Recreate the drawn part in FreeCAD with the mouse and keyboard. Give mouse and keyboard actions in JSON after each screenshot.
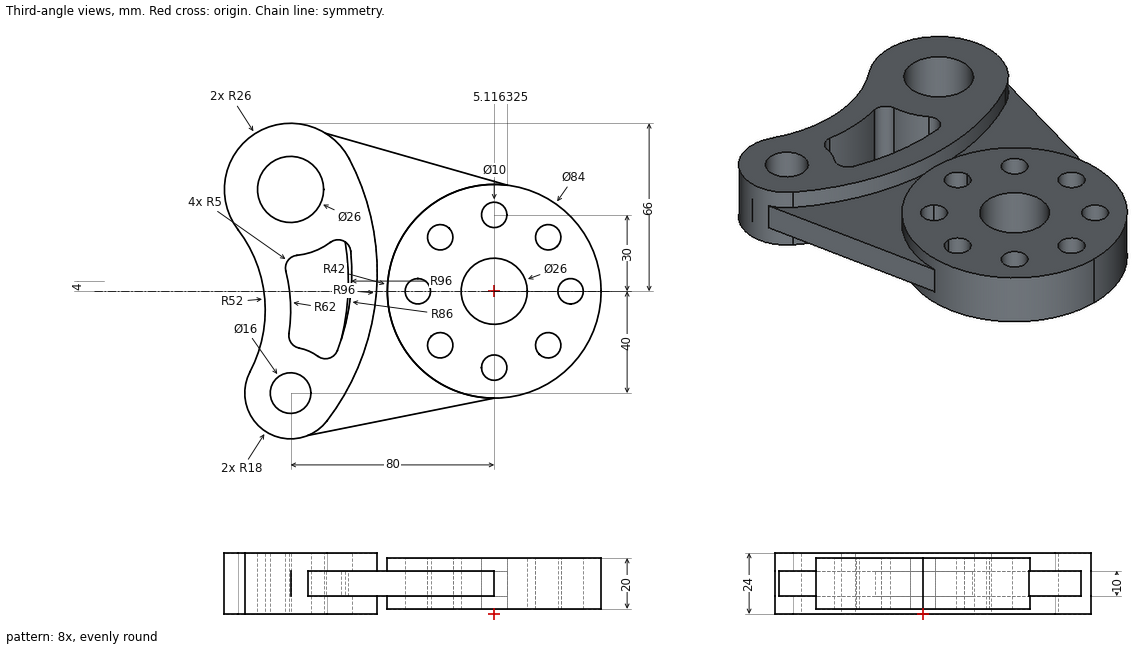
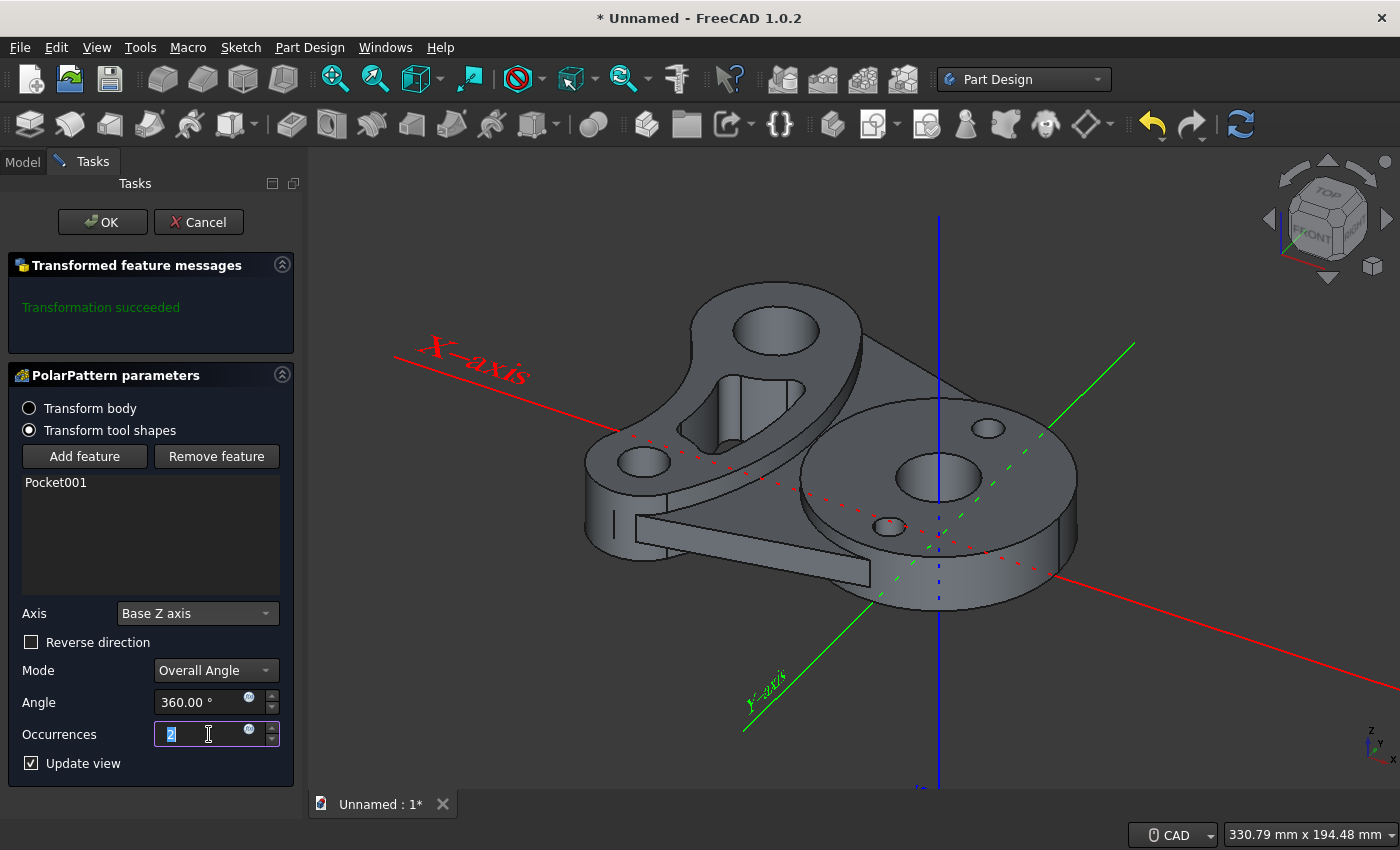
{"action": "type", "text": "8"}
{"action": "key", "text": "Tab"}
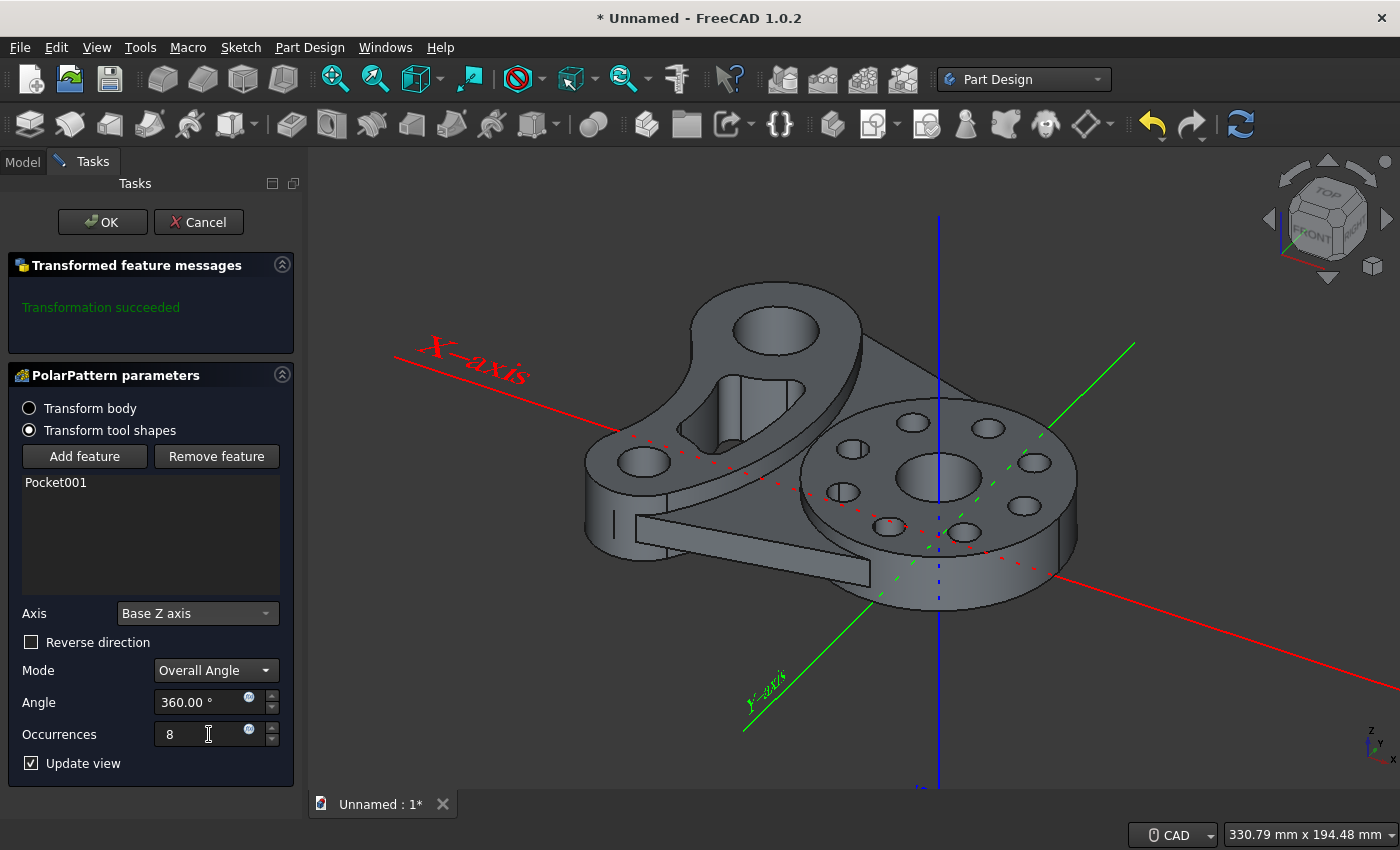
{"action": "left_click", "coordinate": [103, 222]}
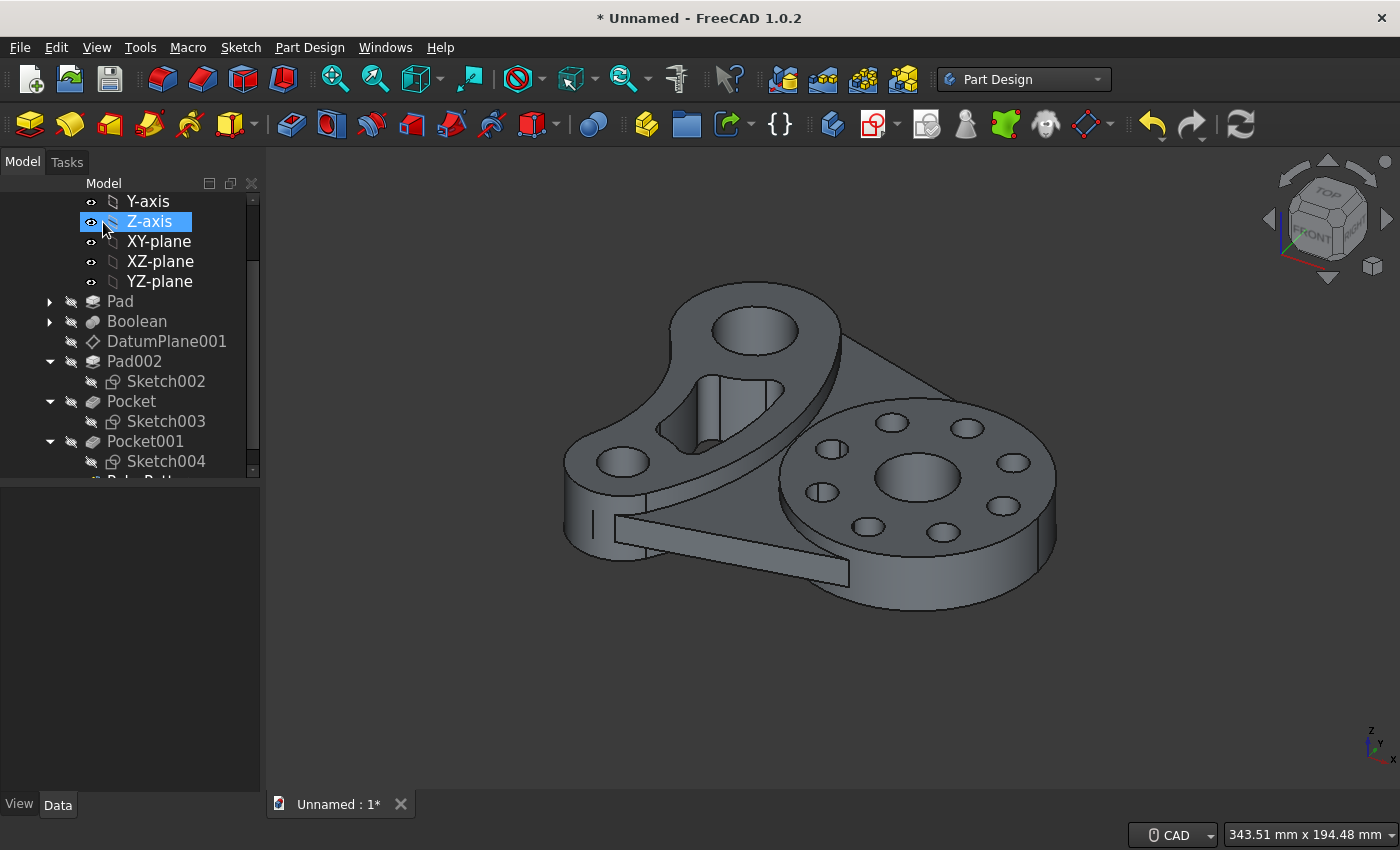
{"action": "key", "text": "0"}